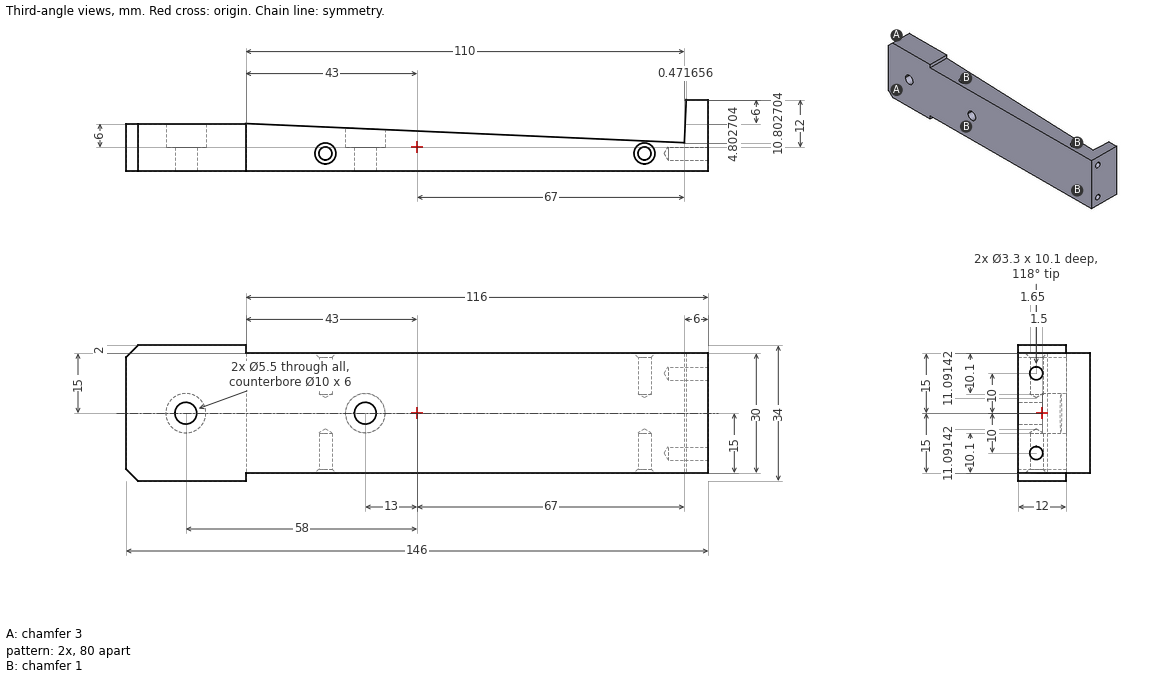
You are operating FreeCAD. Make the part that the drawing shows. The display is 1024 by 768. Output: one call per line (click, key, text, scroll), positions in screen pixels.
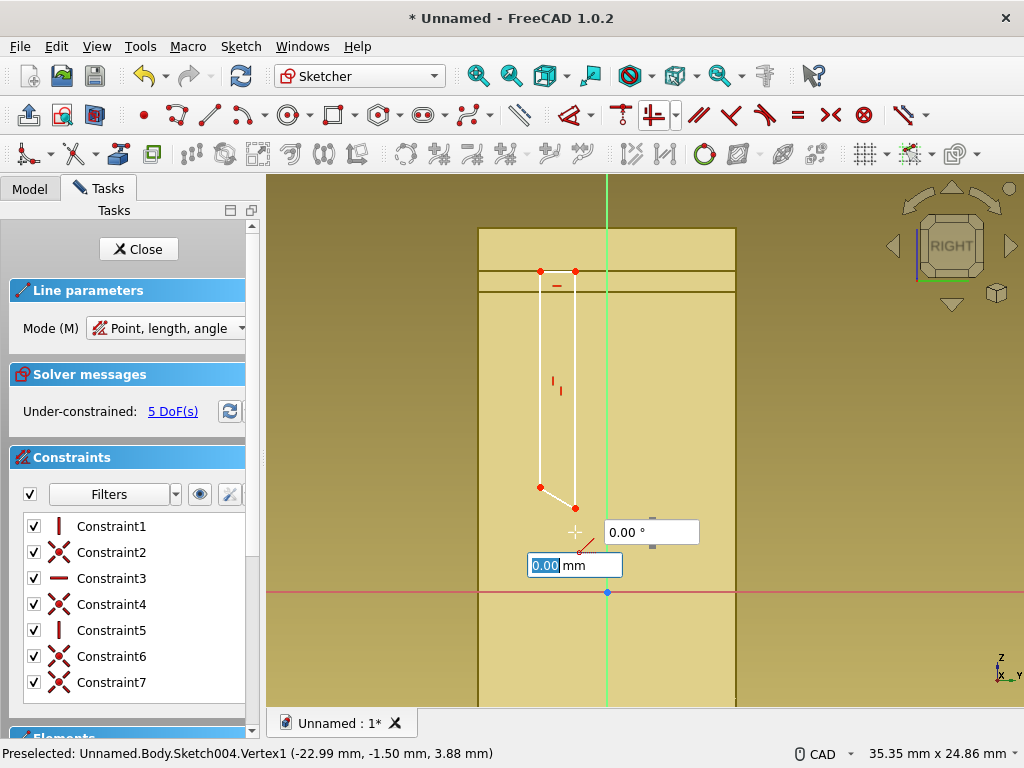
scroll(575, 604, up, 2)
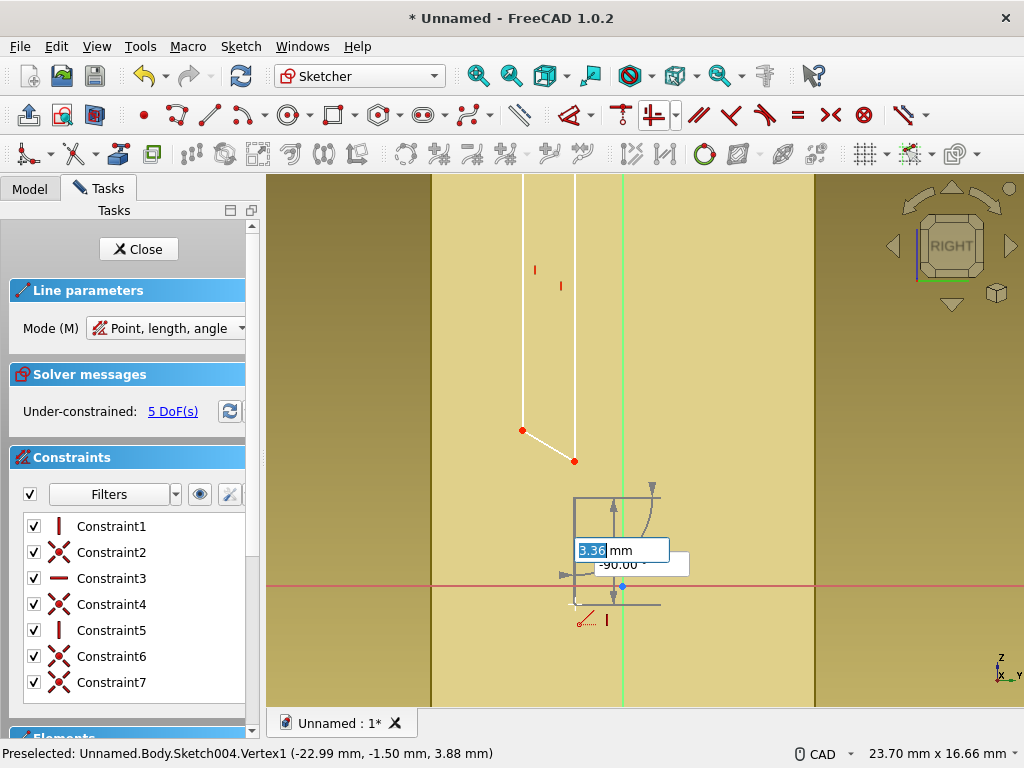
click(575, 603)
key(Escape)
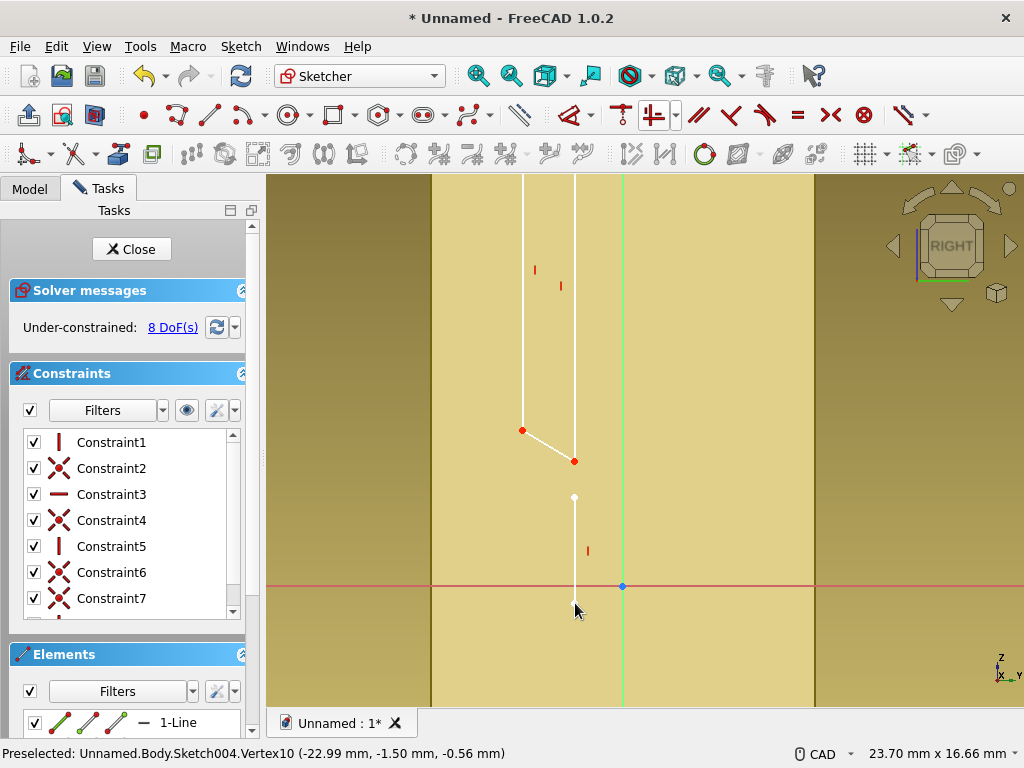
click(575, 530)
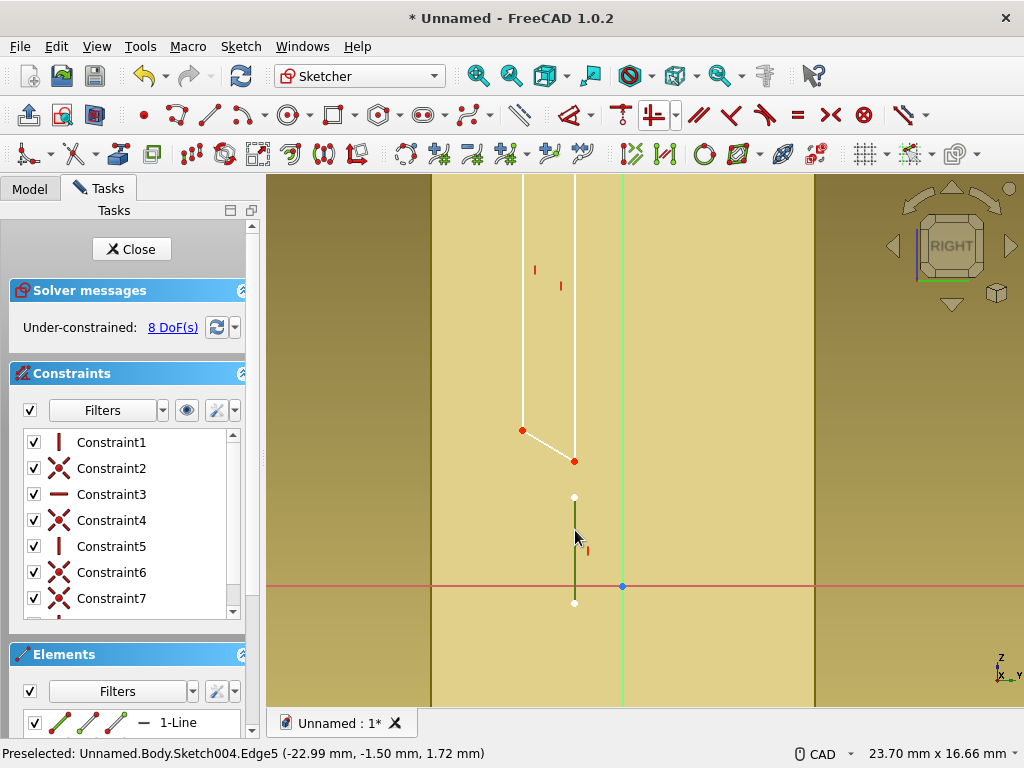
key(g)
key(n)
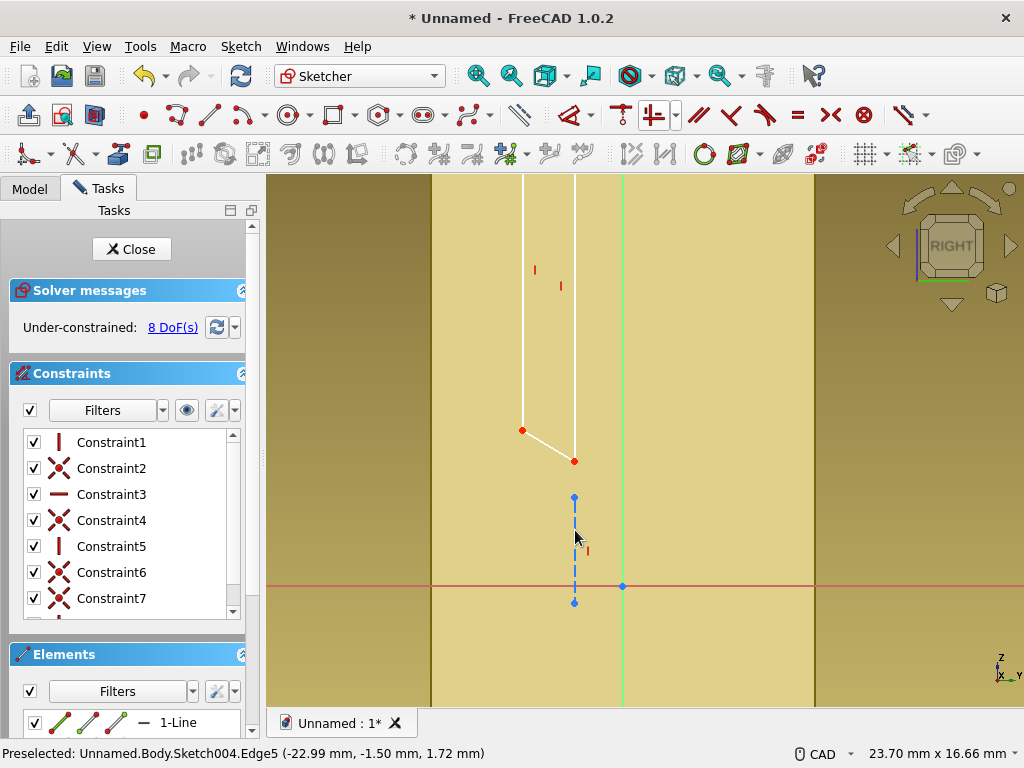
click(568, 116)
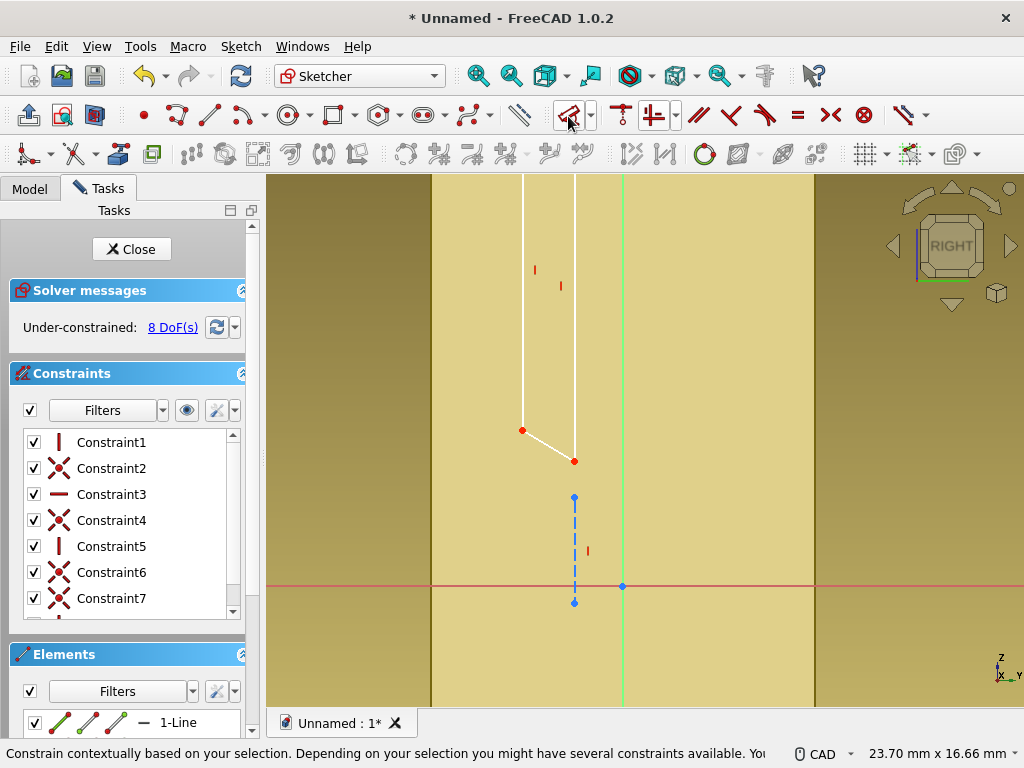
scroll(585, 615, down, 2)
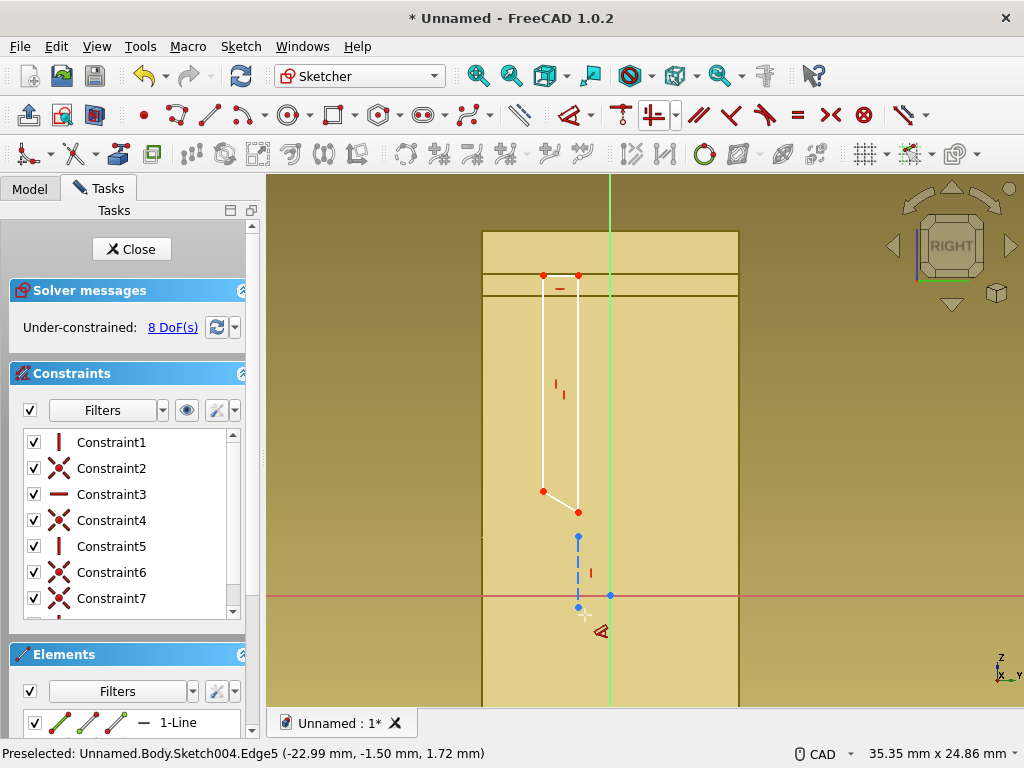
click(578, 276)
click(644, 436)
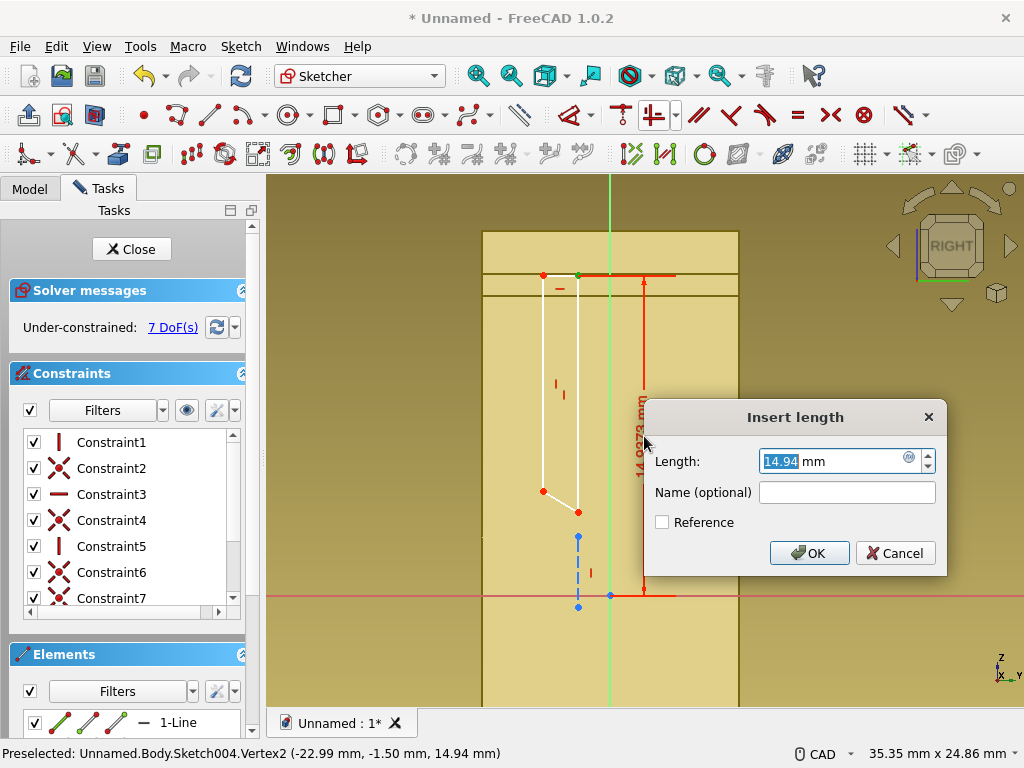
text(15)
key(Return)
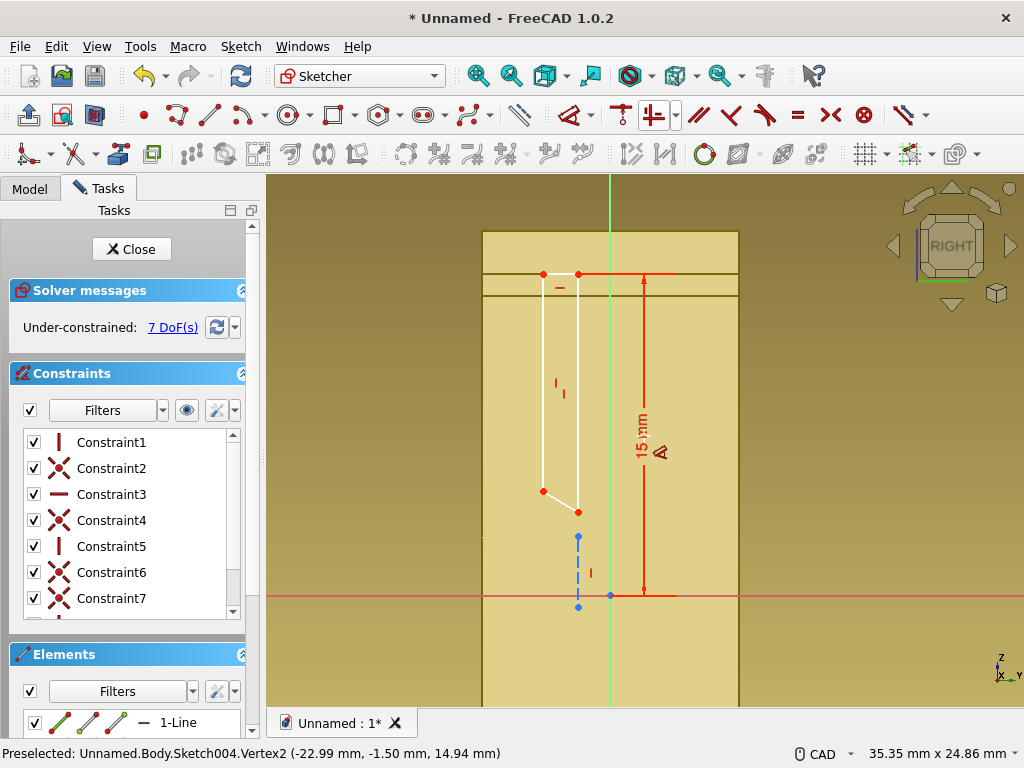
scroll(568, 274, up, 2)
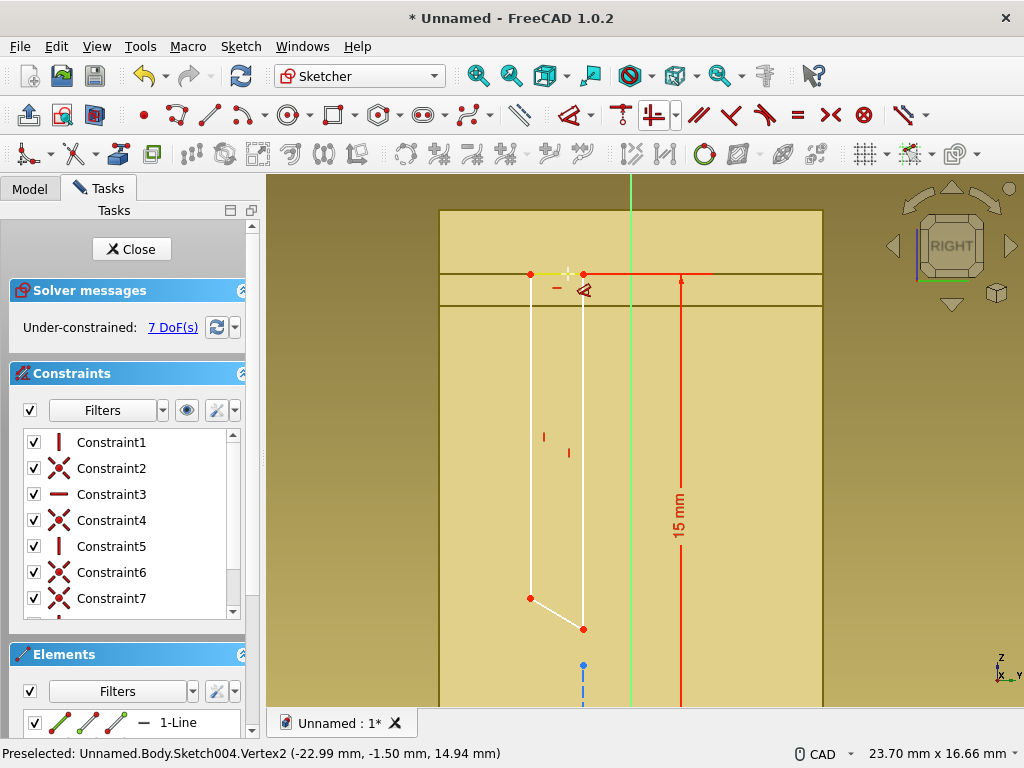
click(568, 274)
click(557, 240)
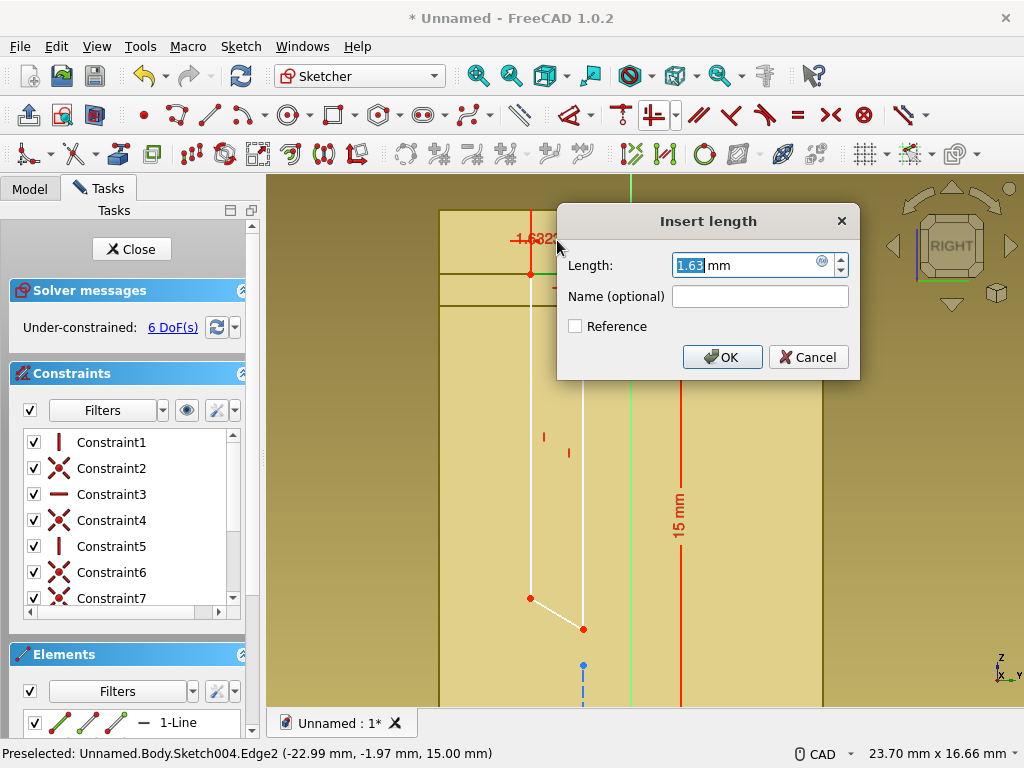
text(1.65)
key(Return)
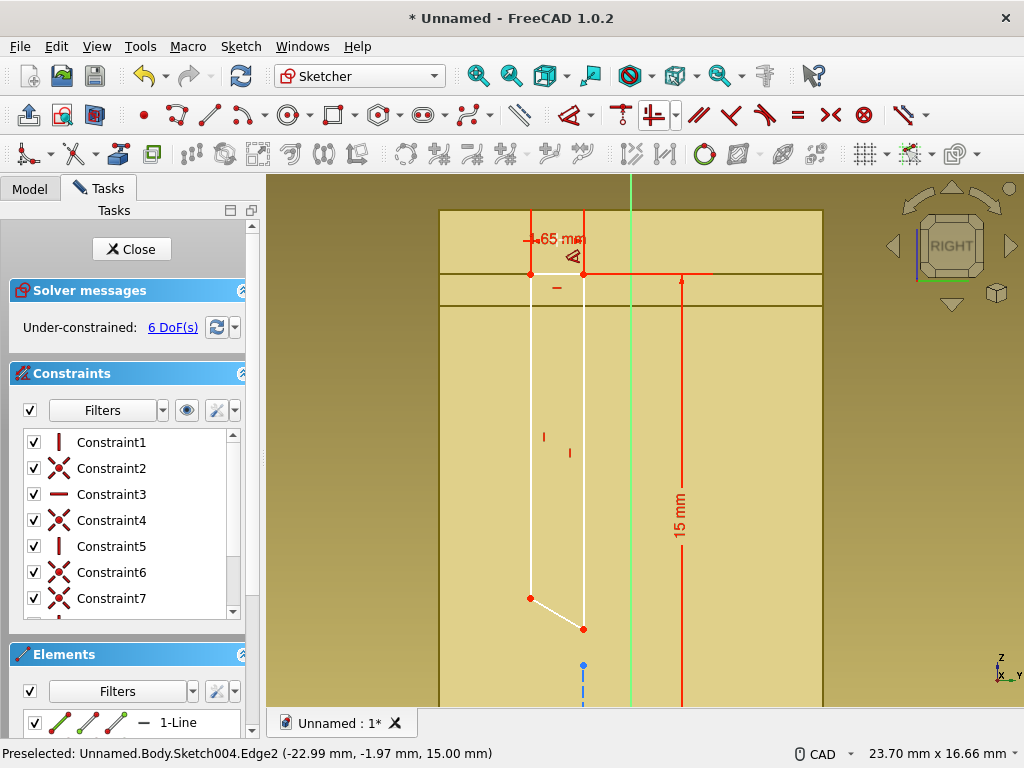
click(531, 372)
click(497, 436)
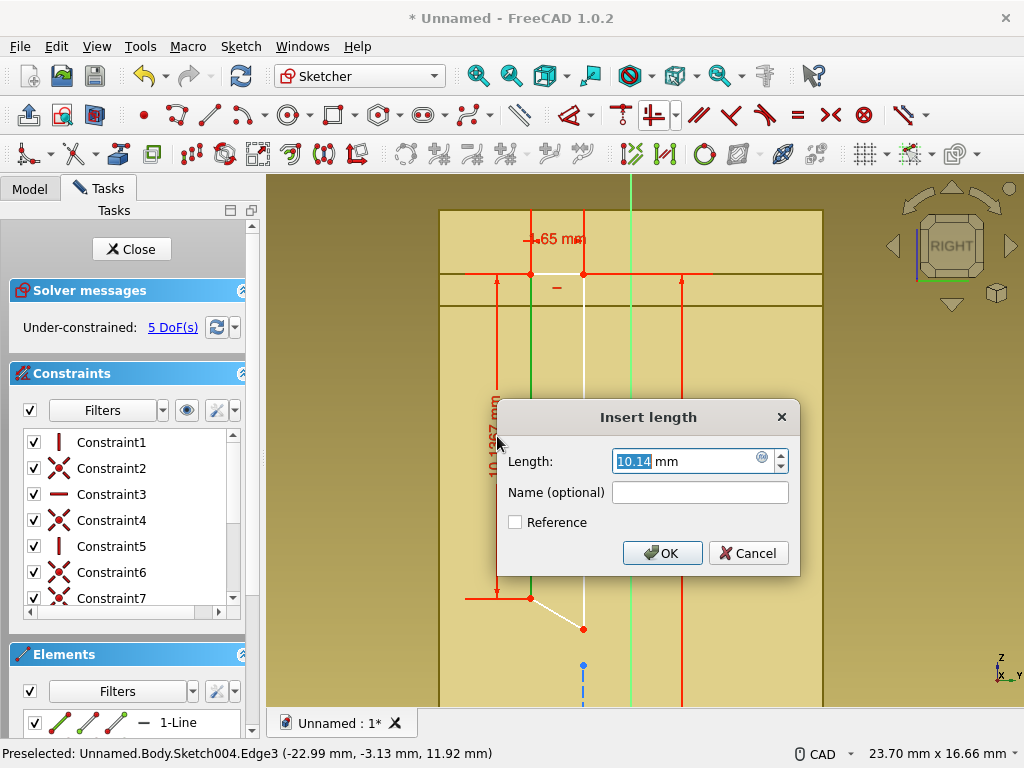
text(10.1)
key(Return)